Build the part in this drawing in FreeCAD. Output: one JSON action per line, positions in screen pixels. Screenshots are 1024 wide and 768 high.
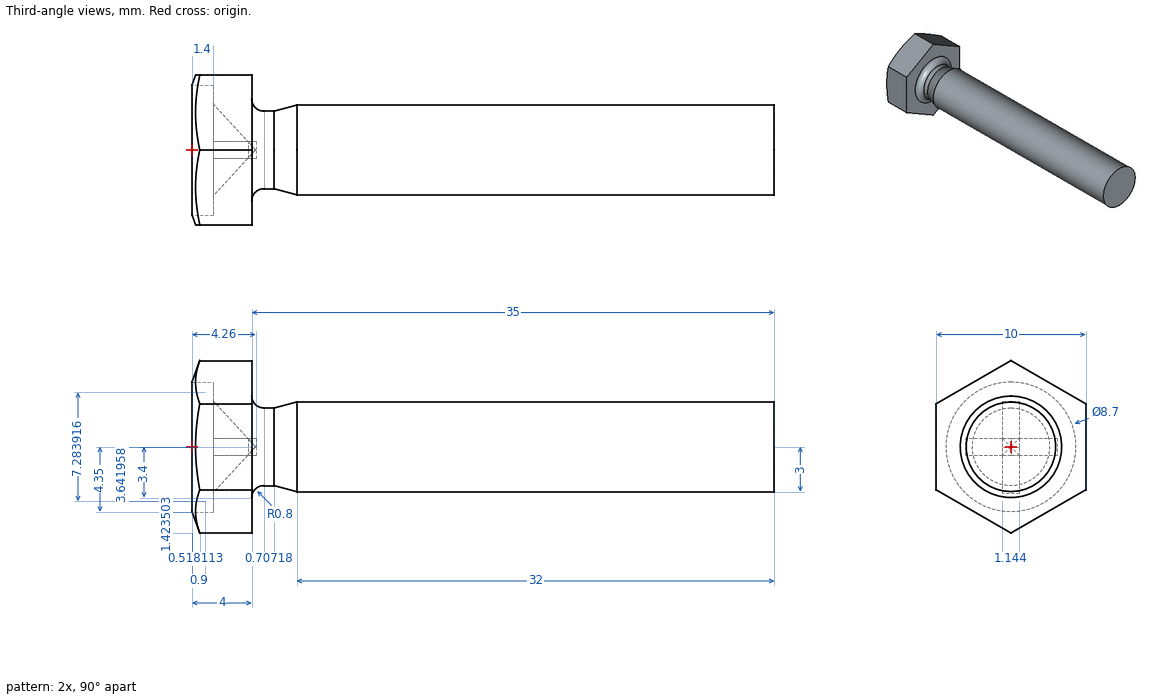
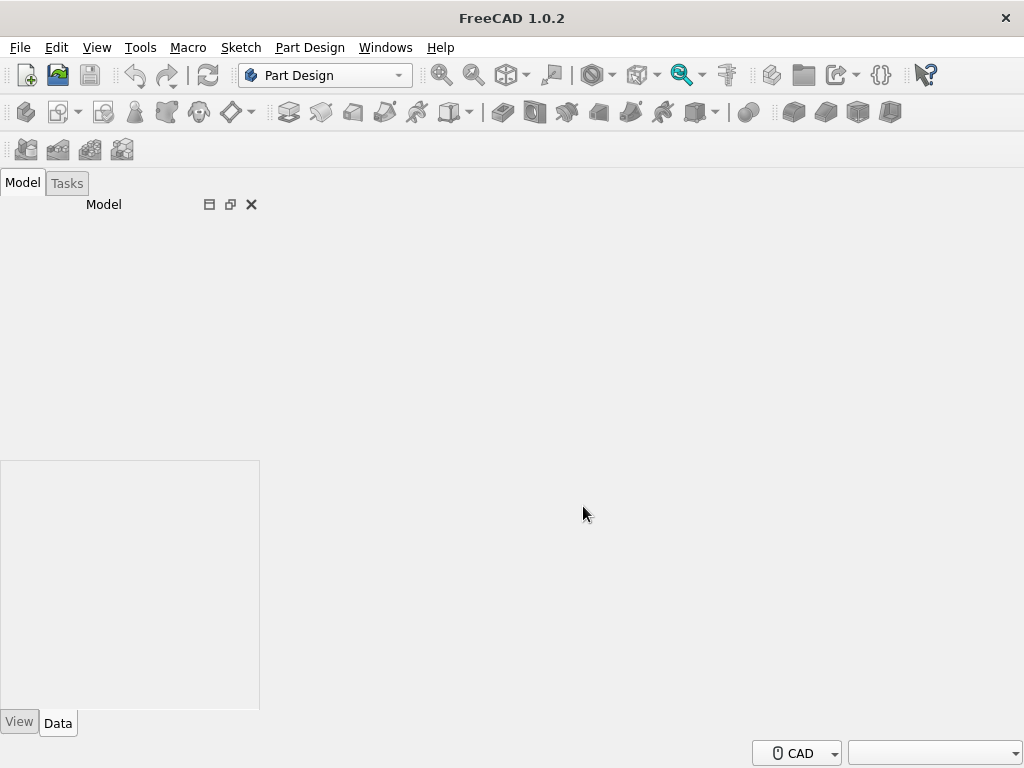
{"action": "key", "text": "ctrl+n"}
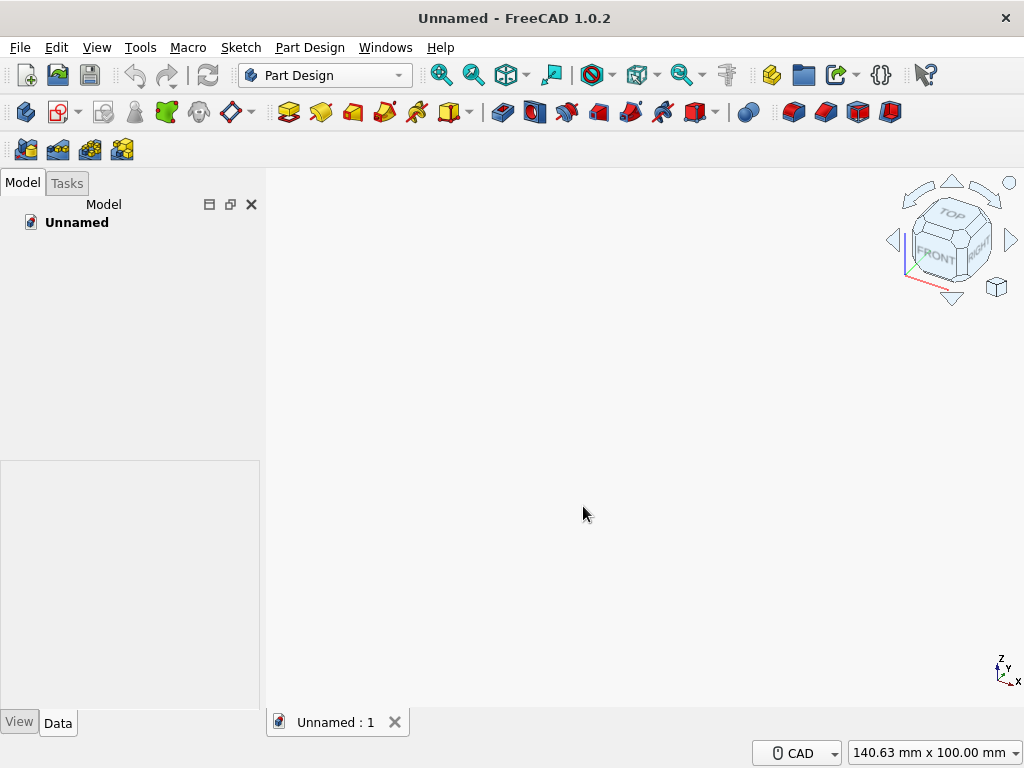
{"action": "left_click", "coordinate": [58, 112]}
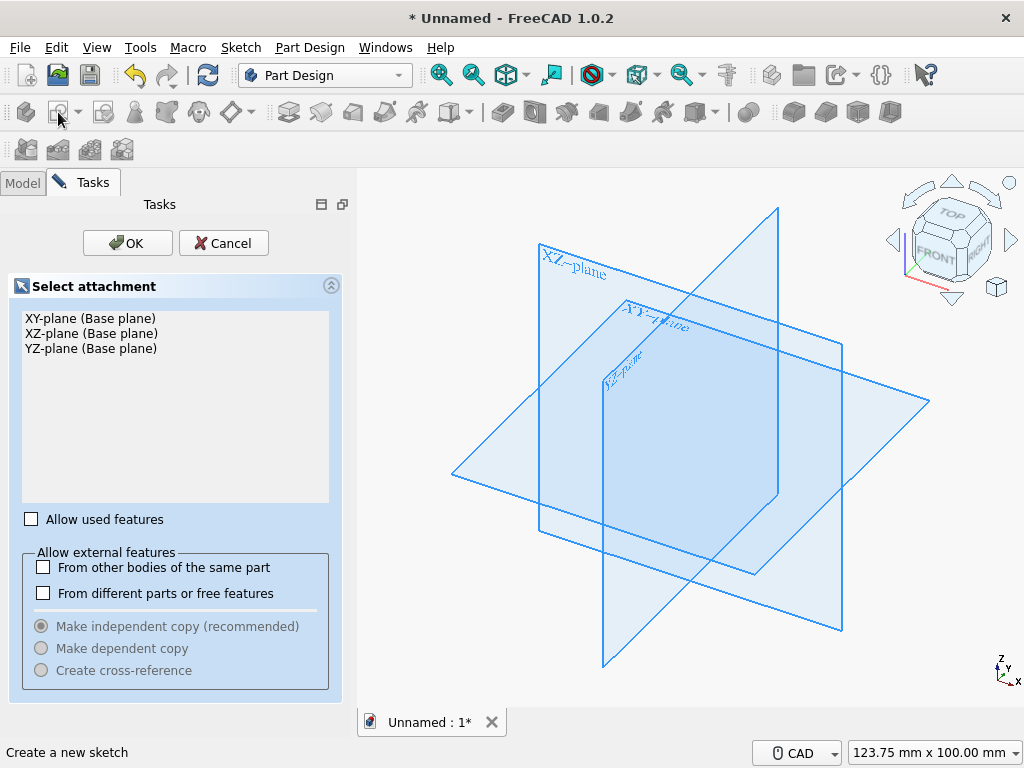
{"action": "left_click", "coordinate": [82, 348]}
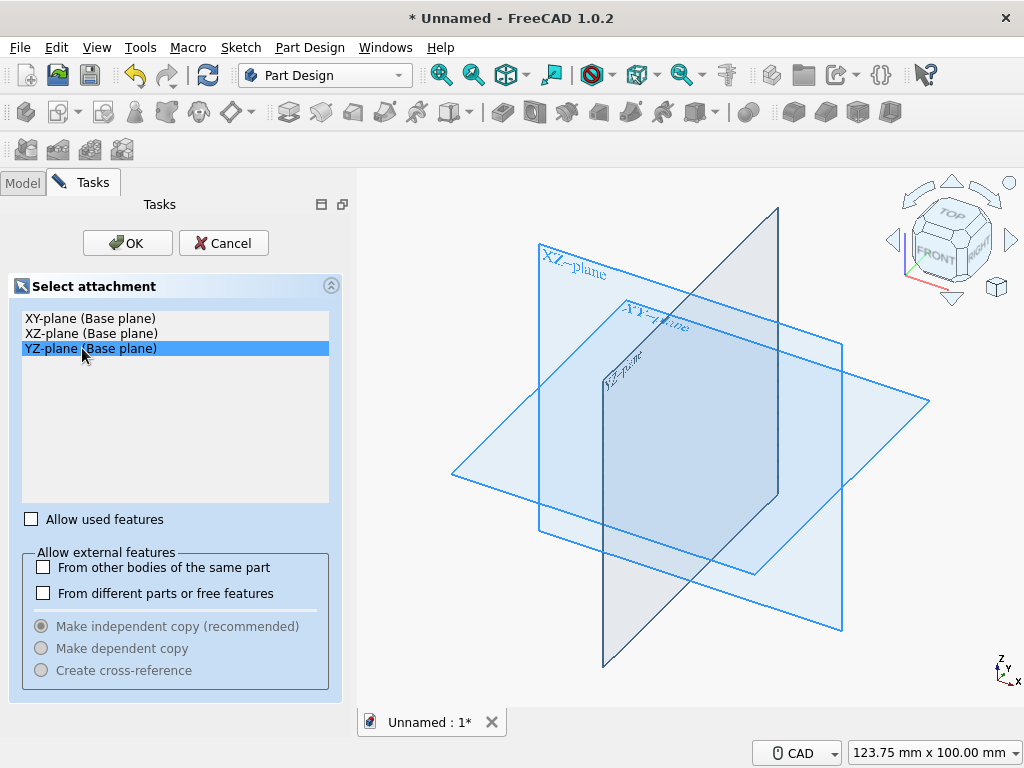
{"action": "left_click", "coordinate": [128, 243]}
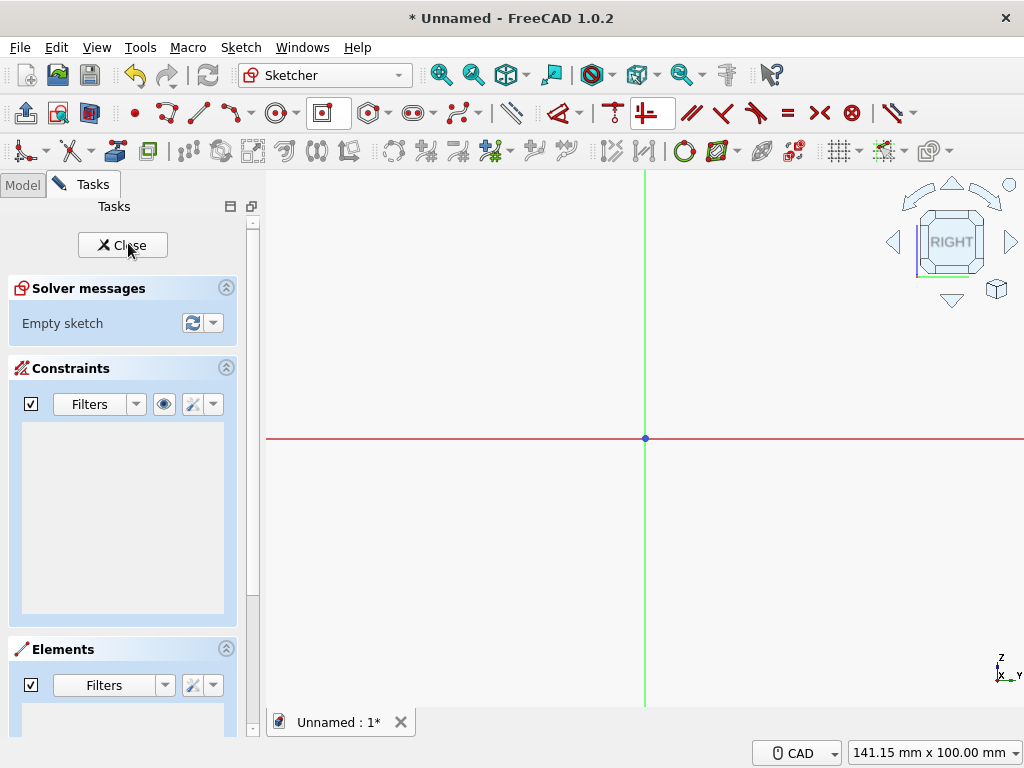
{"action": "scroll", "coordinate": [659, 438], "scroll_direction": "up", "scroll_amount": 9}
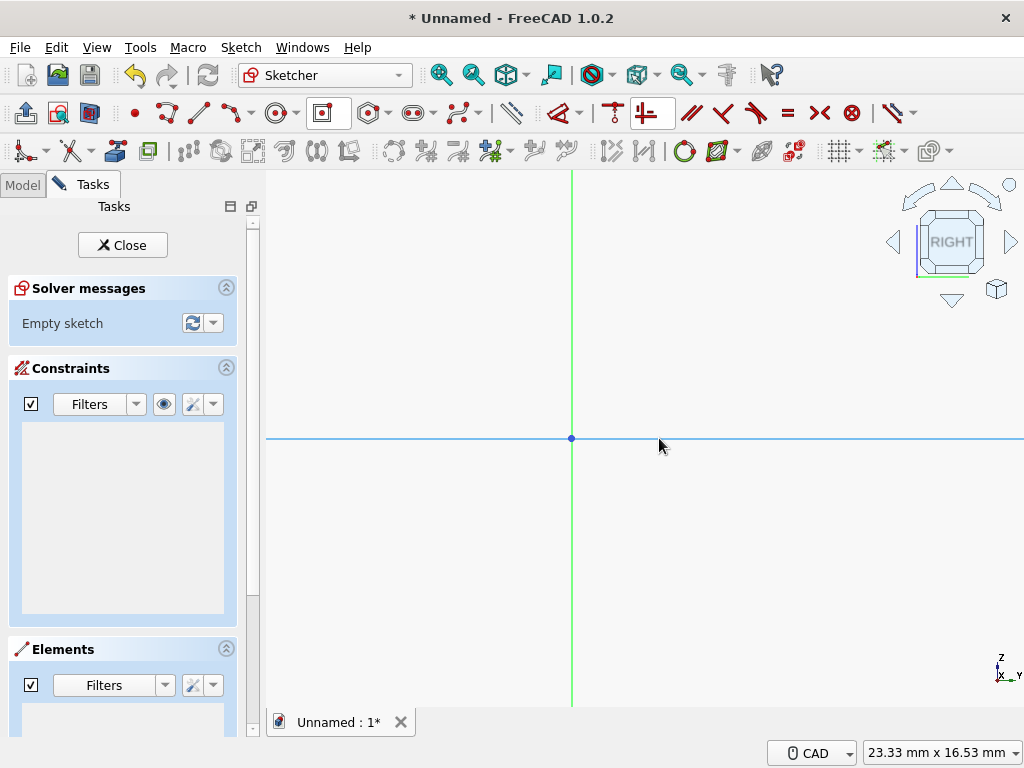
{"action": "left_click", "coordinate": [368, 114]}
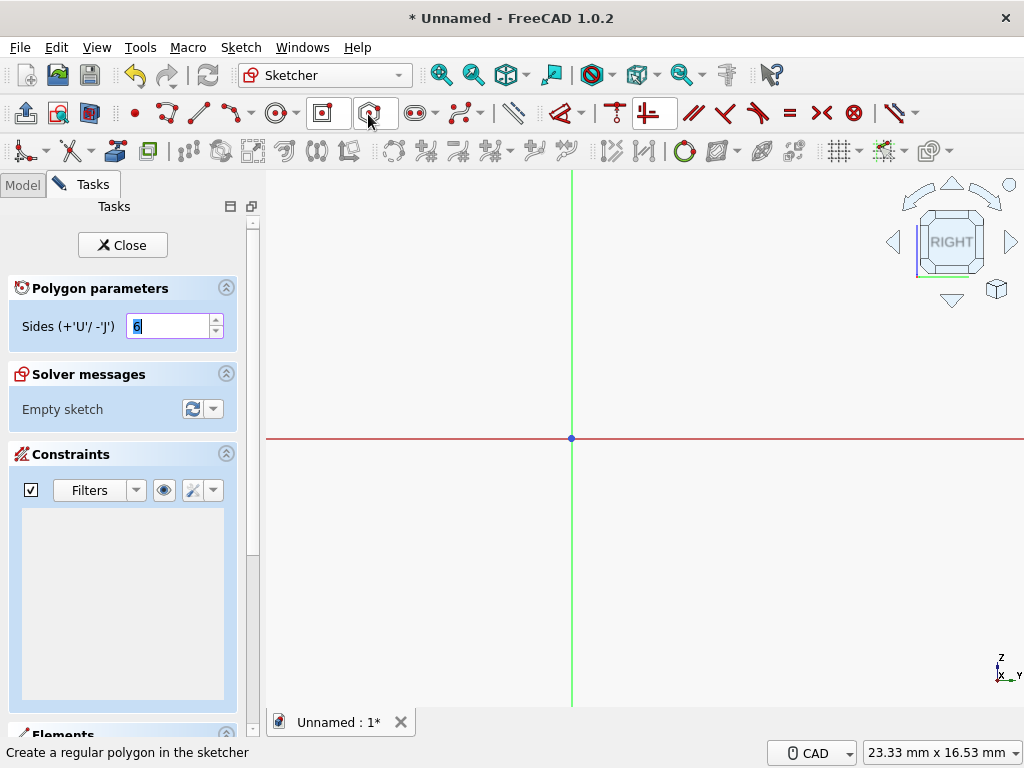
{"action": "left_click", "coordinate": [572, 438]}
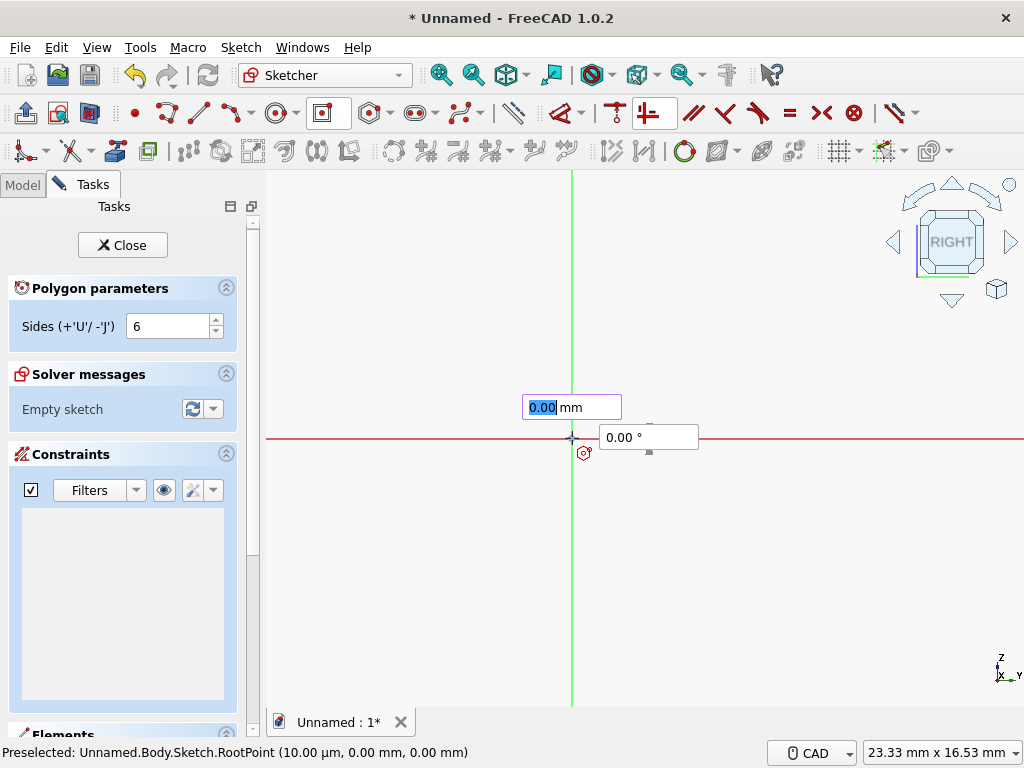
{"action": "left_click", "coordinate": [572, 626]}
{"action": "key", "text": "Escape"}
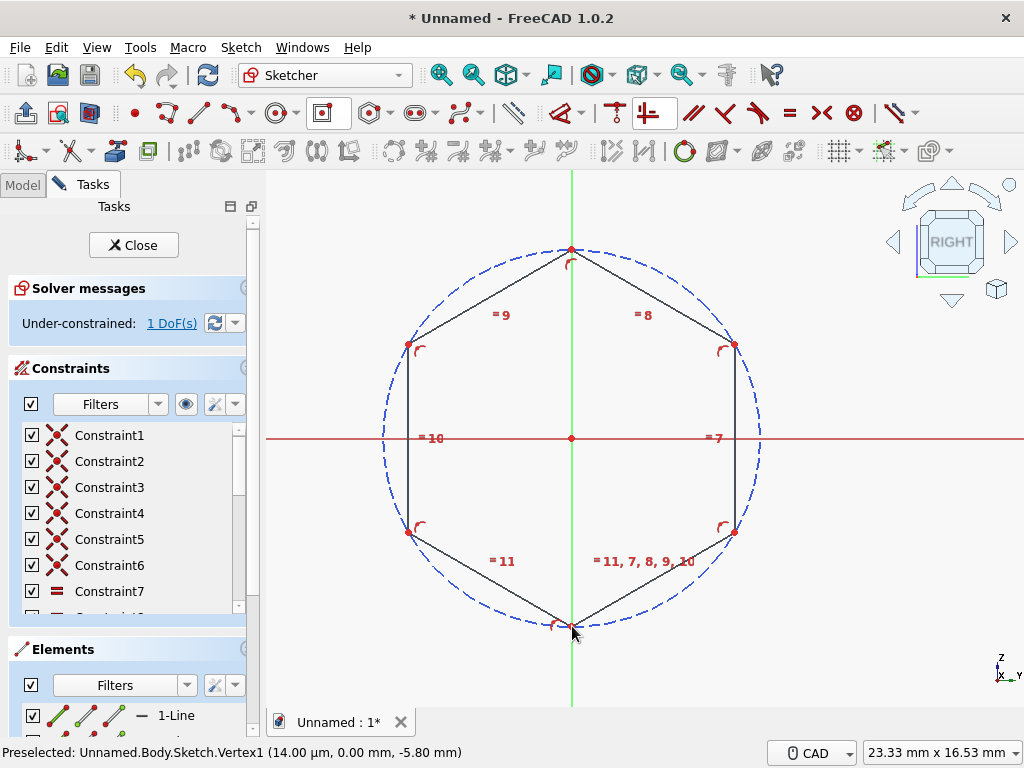
{"action": "left_click", "coordinate": [408, 344]}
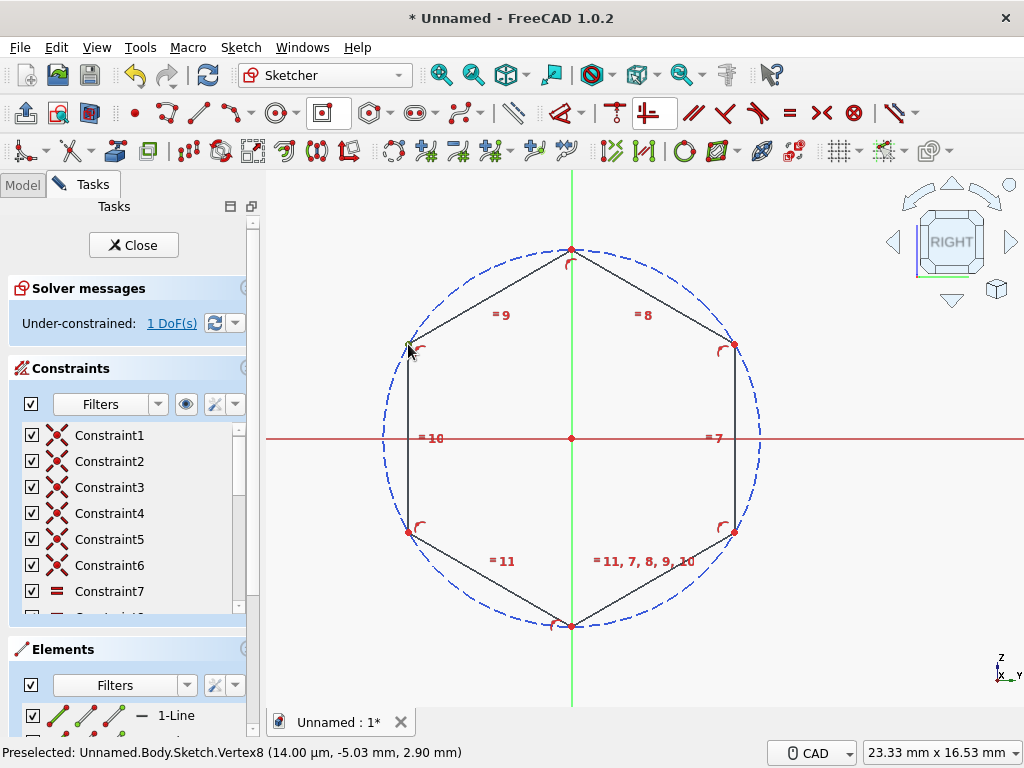
{"action": "left_click", "coordinate": [735, 533]}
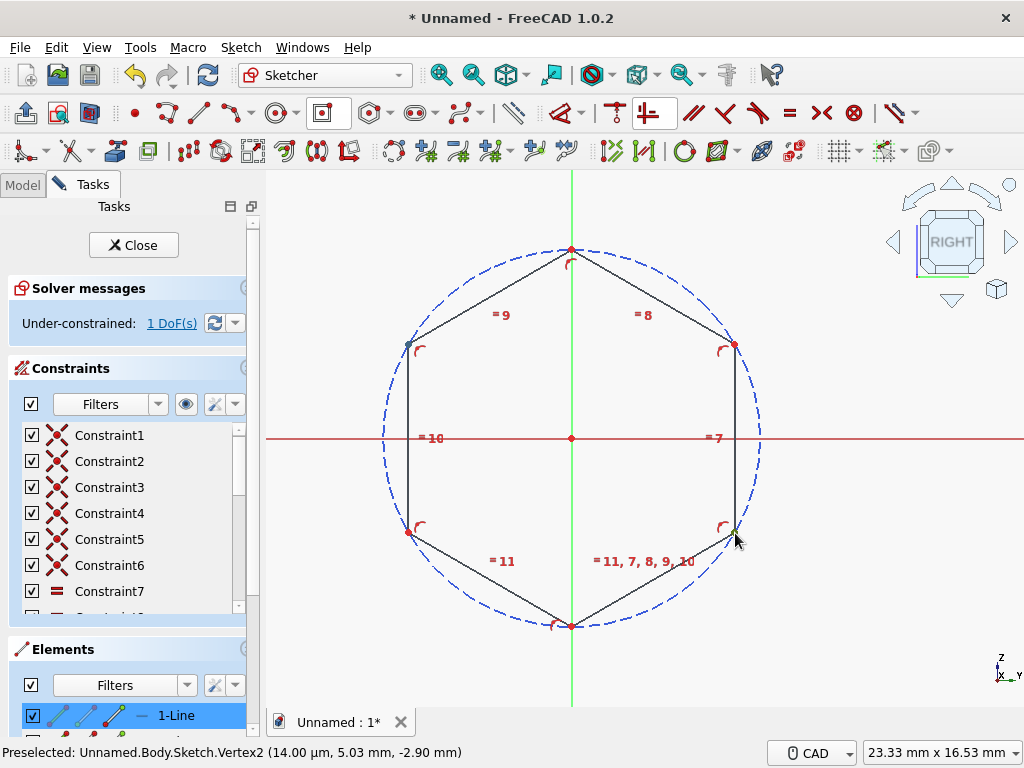
{"action": "key", "text": "l"}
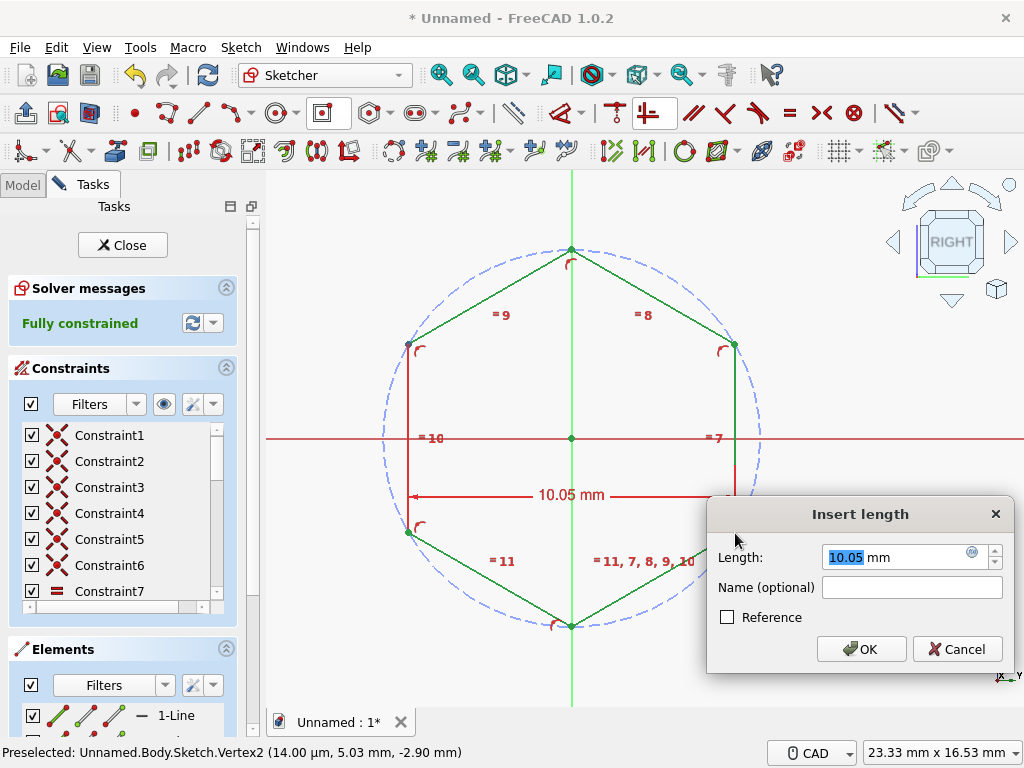
{"action": "type", "text": "10"}
{"action": "key", "text": "Return"}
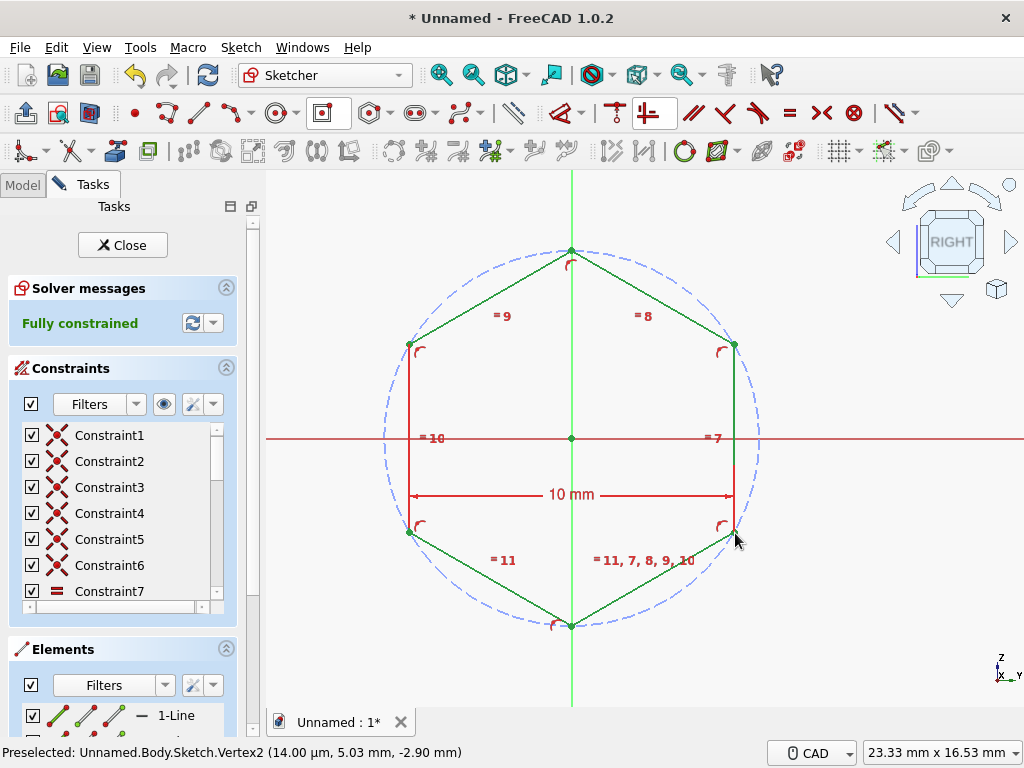
{"action": "left_click", "coordinate": [123, 245]}